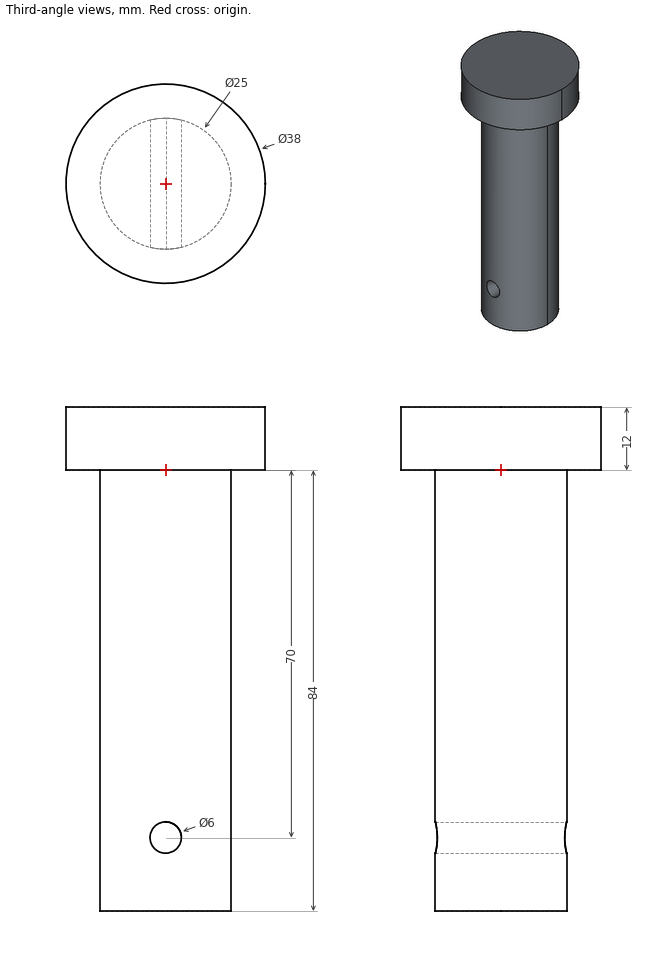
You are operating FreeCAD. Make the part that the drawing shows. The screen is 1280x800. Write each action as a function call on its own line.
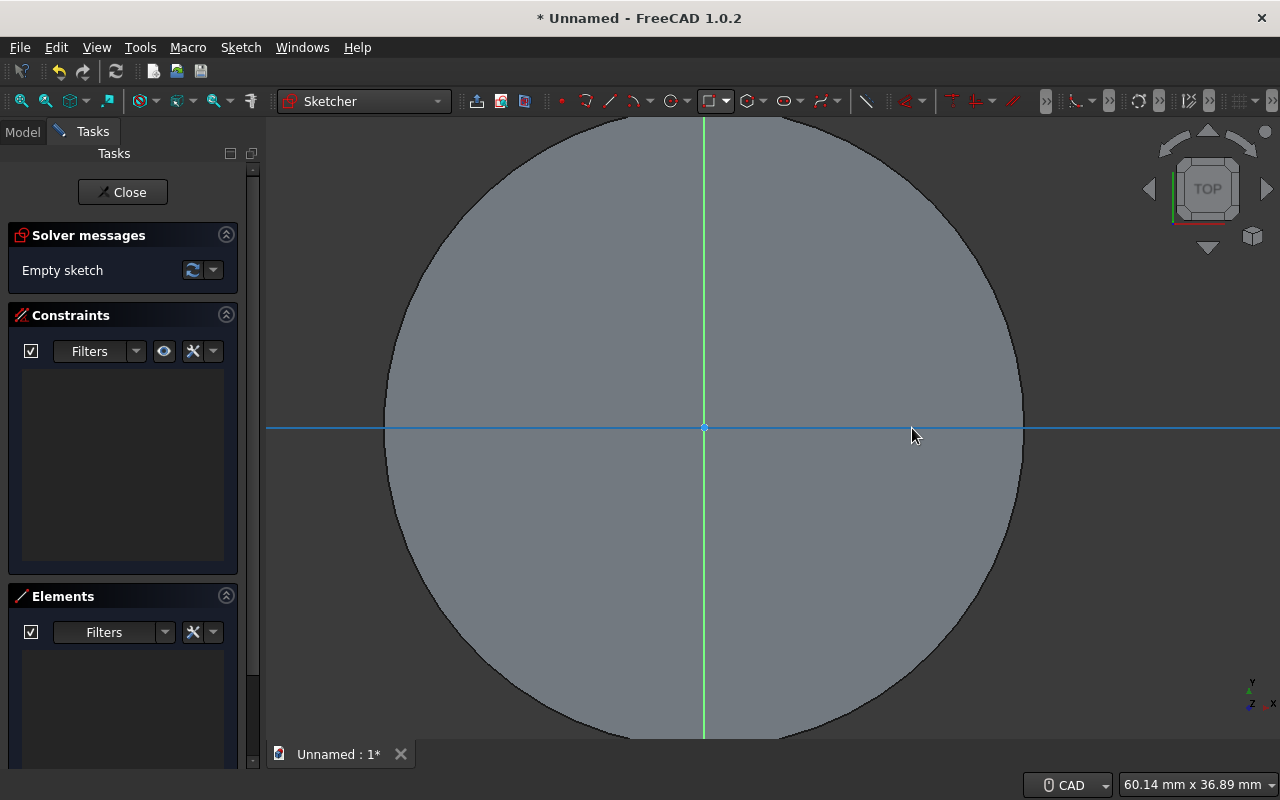
click(672, 102)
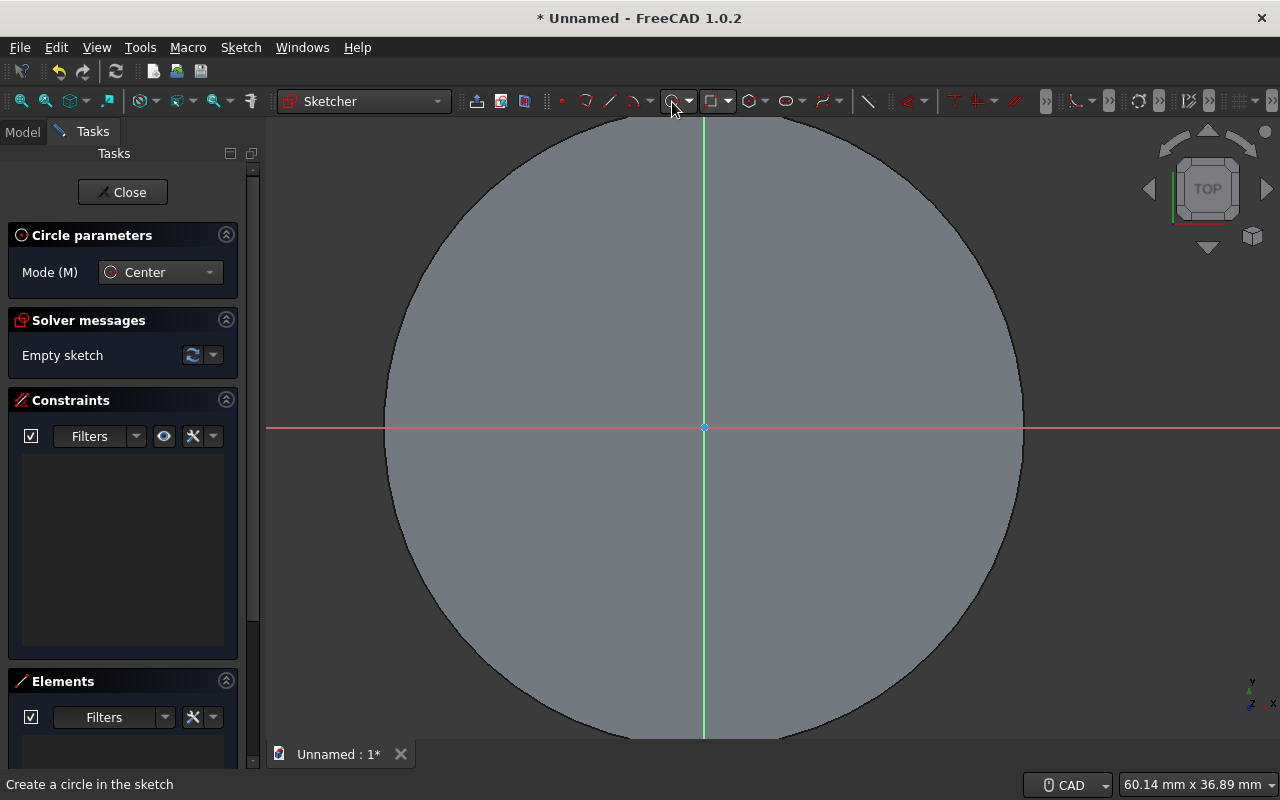
click(704, 428)
click(853, 279)
key(Escape)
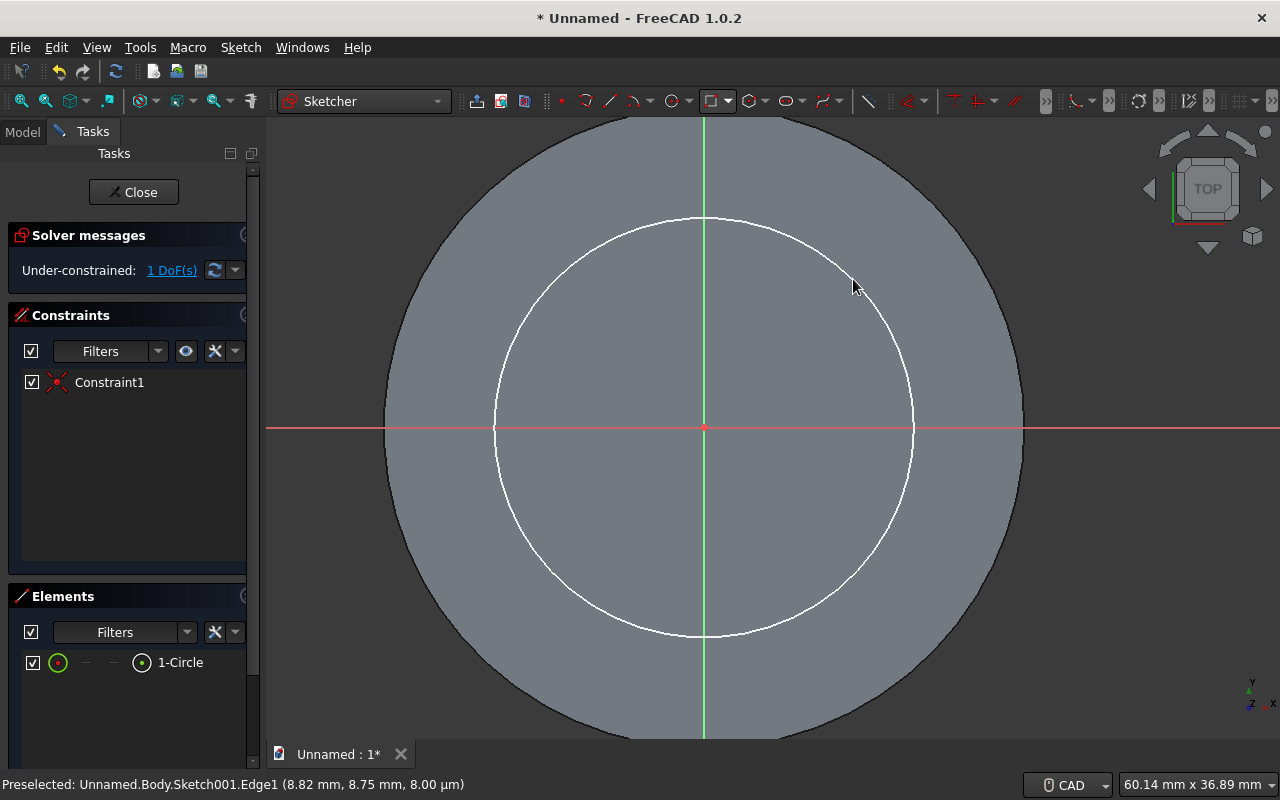
click(908, 102)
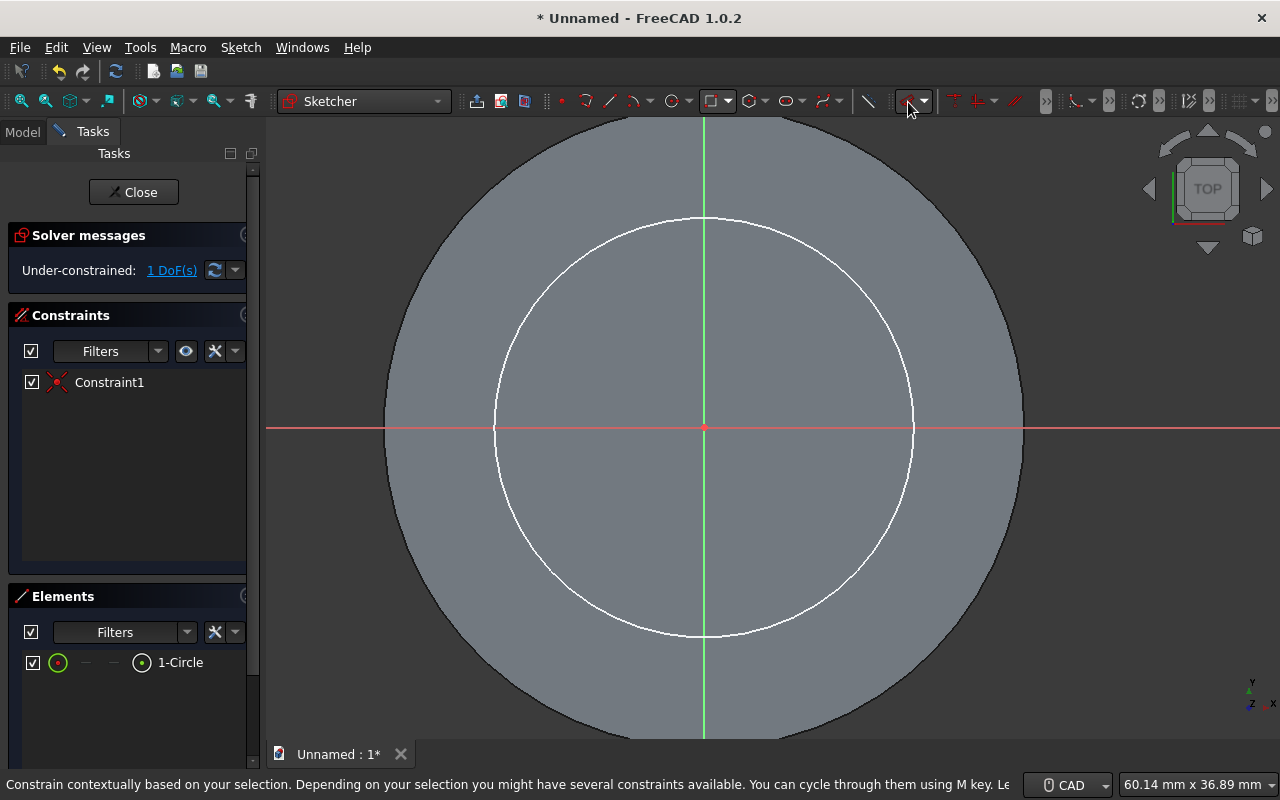
click(852, 279)
click(875, 256)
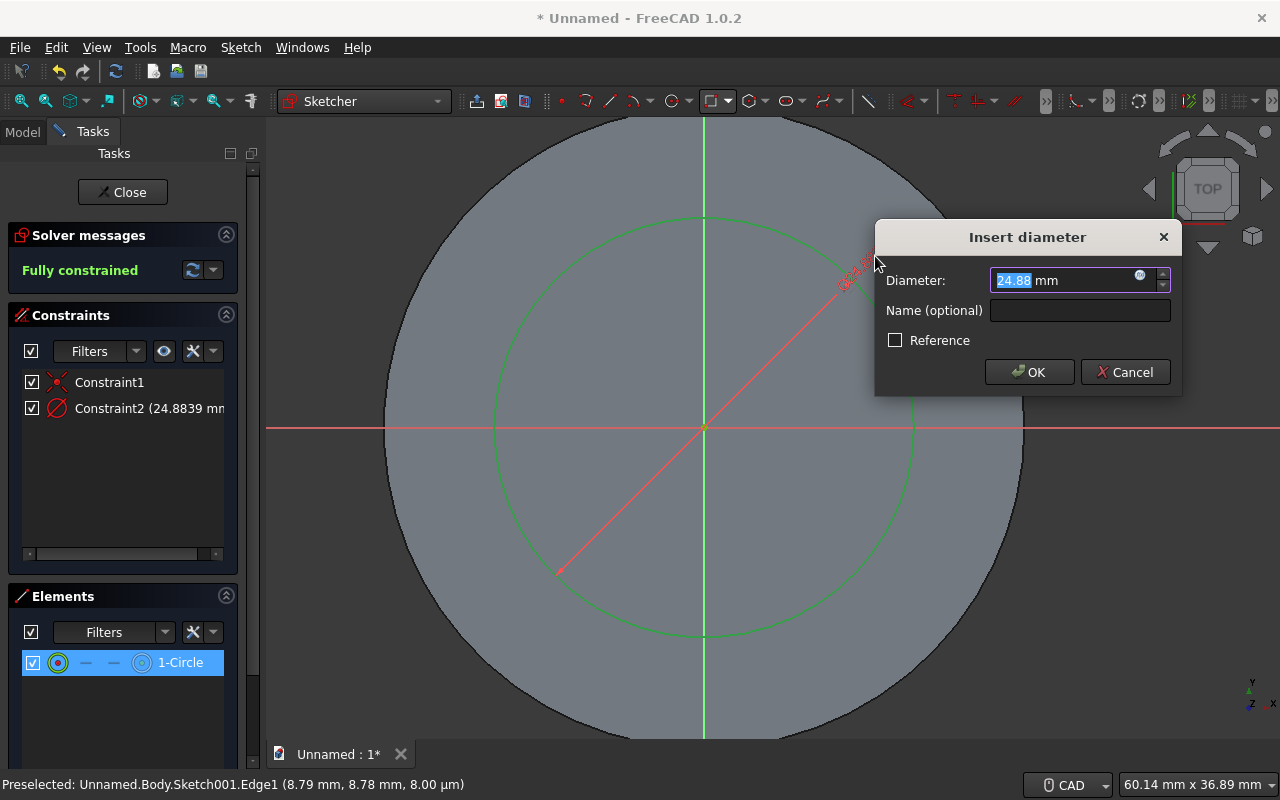
text(25)
key(Return)
key(Escape)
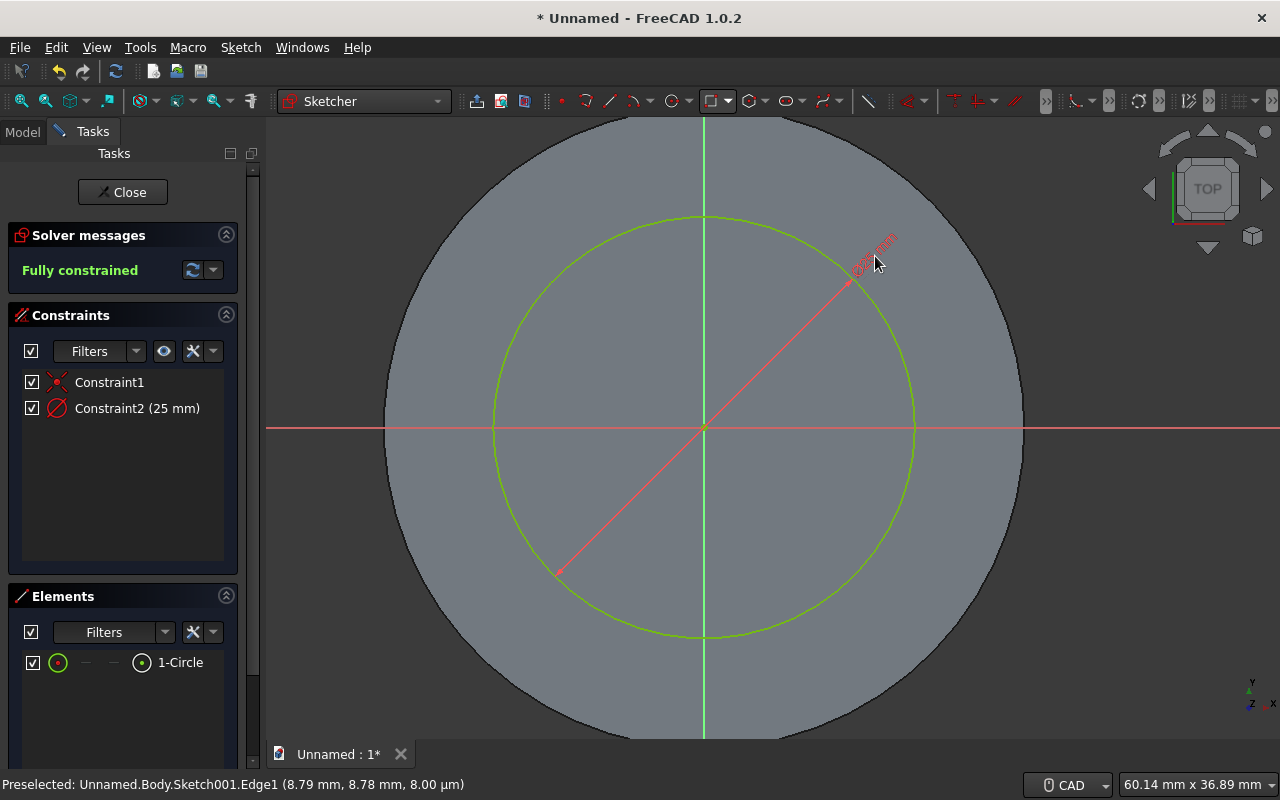
click(123, 192)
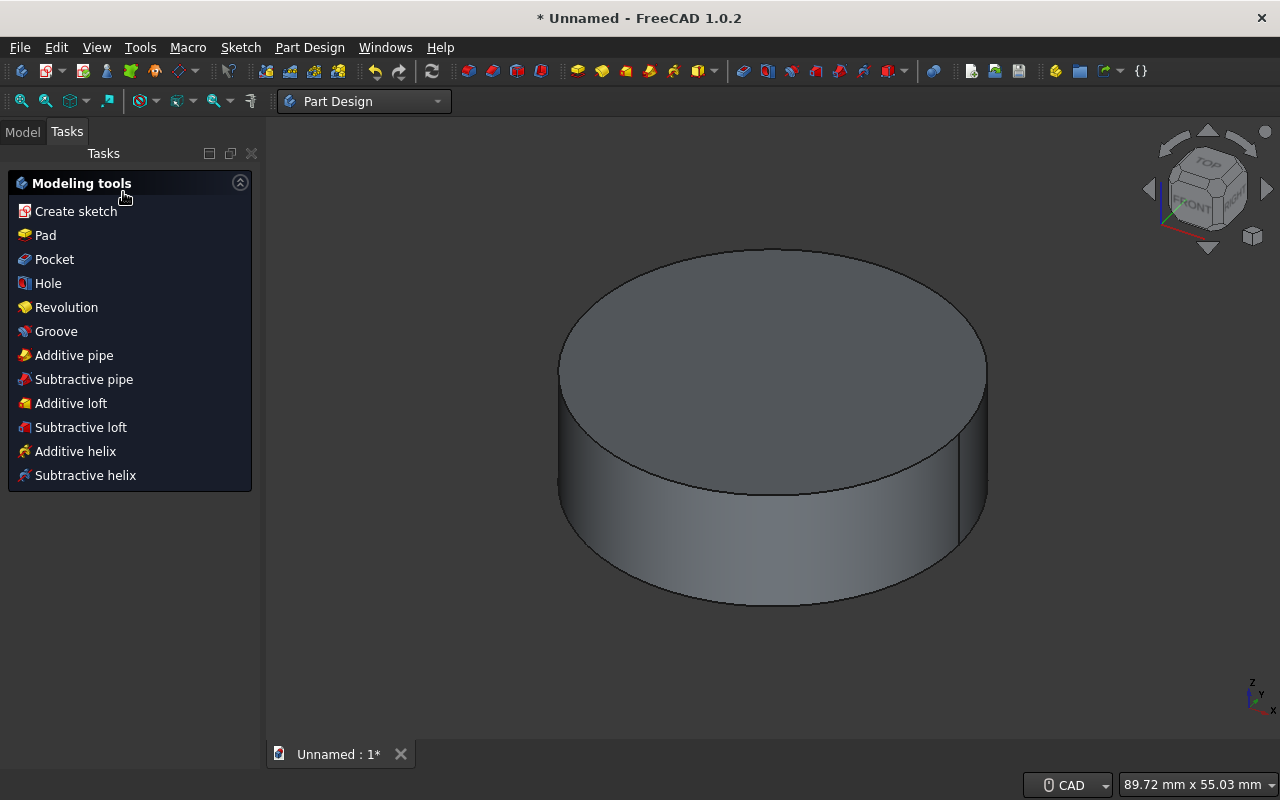
click(578, 72)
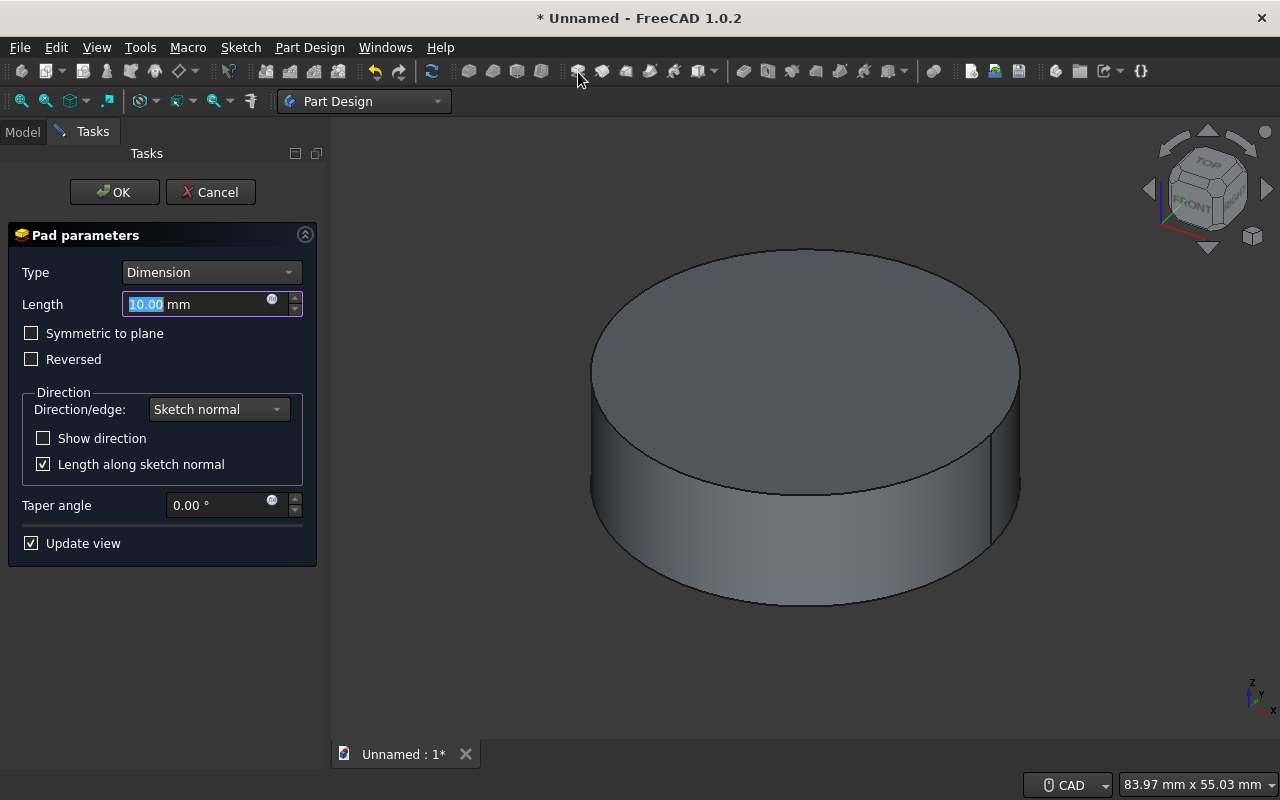
text(84)
key(Tab)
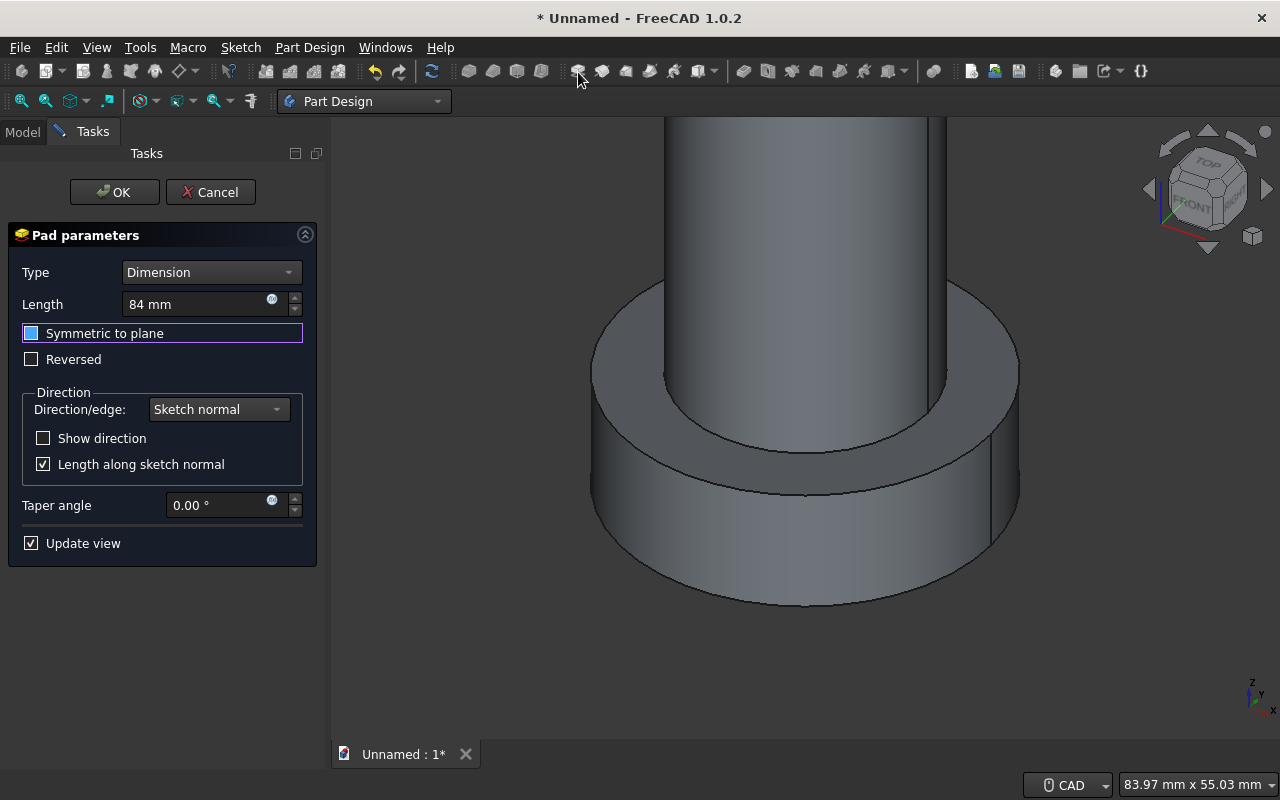
click(30, 359)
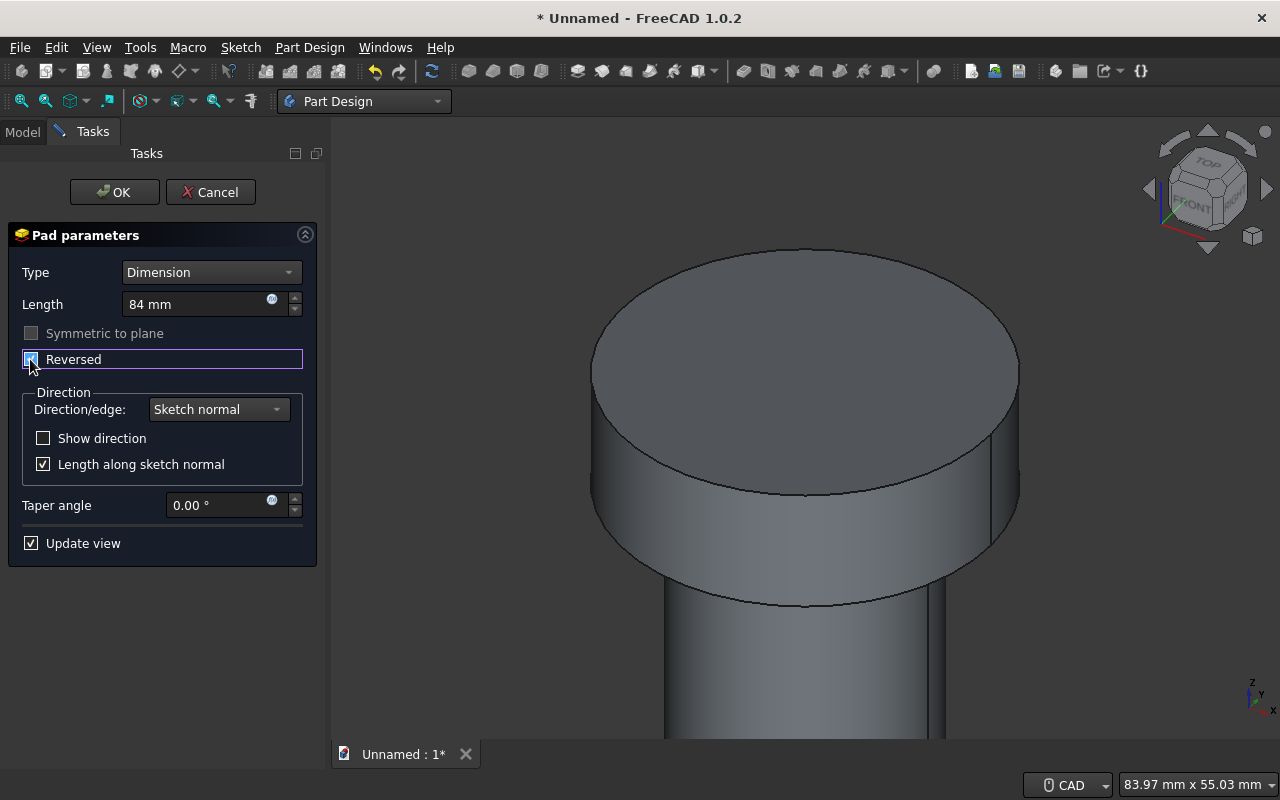
click(115, 192)